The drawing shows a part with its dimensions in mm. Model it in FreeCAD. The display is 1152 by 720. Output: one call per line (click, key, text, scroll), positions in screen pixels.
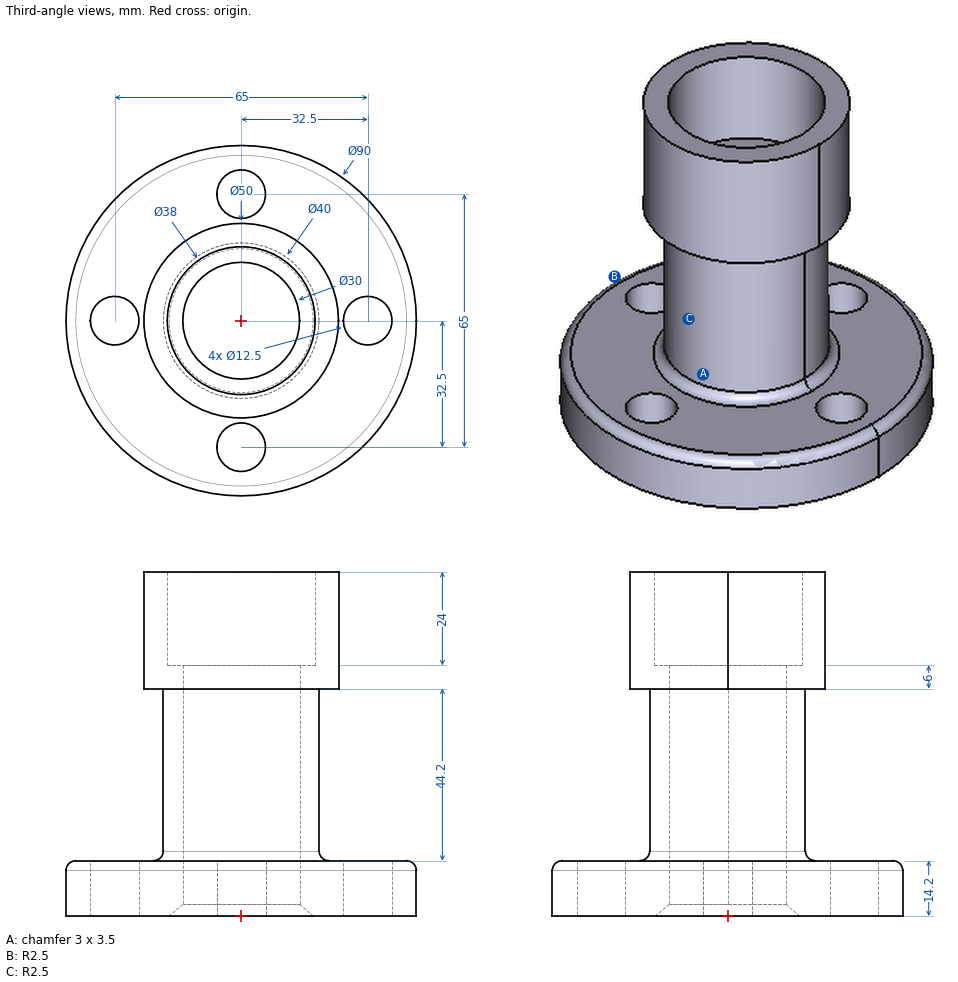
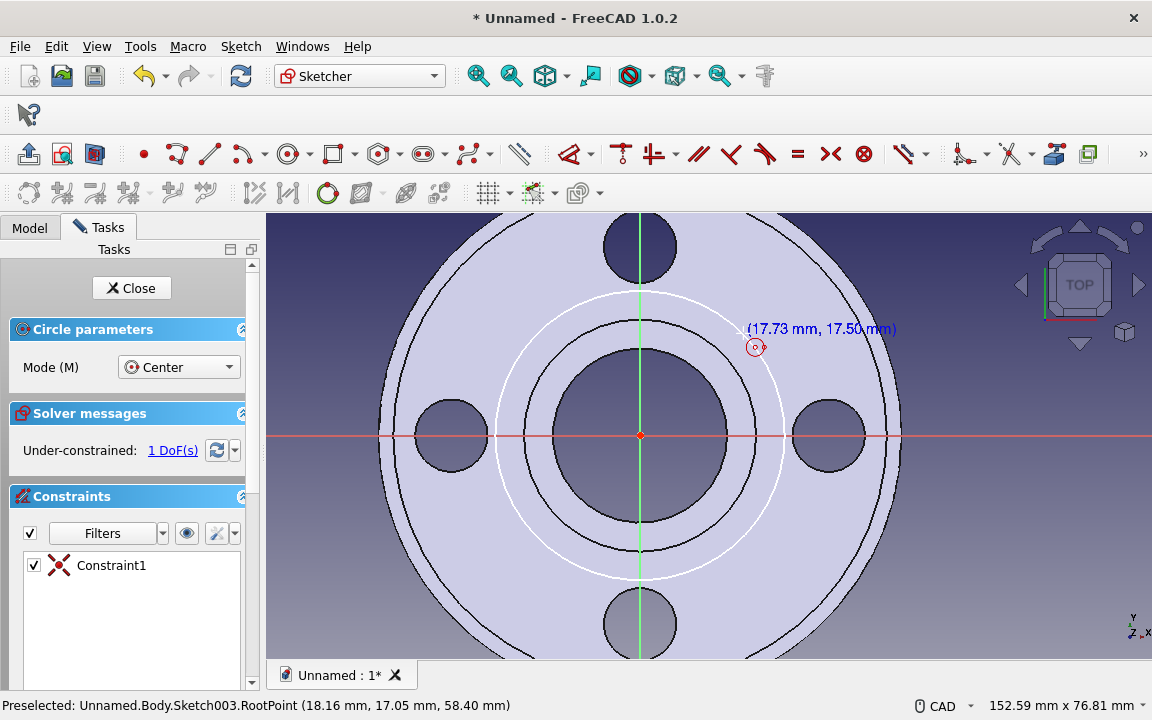
click(640, 436)
click(702, 374)
key(Escape)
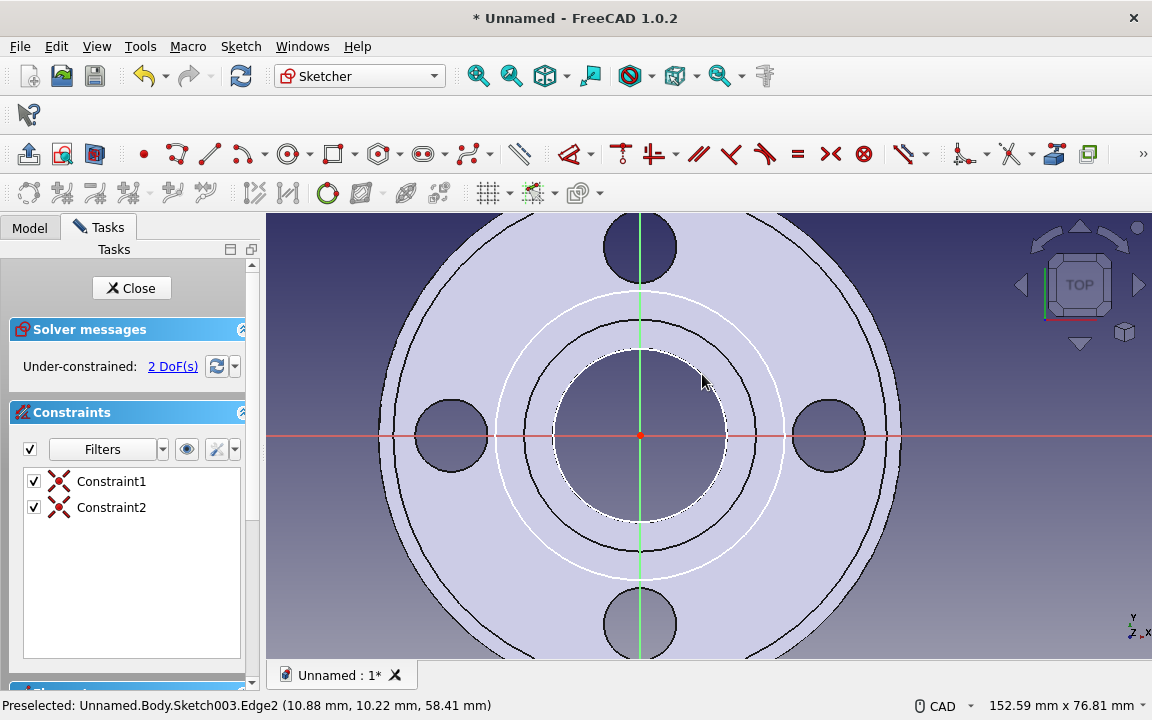
click(568, 154)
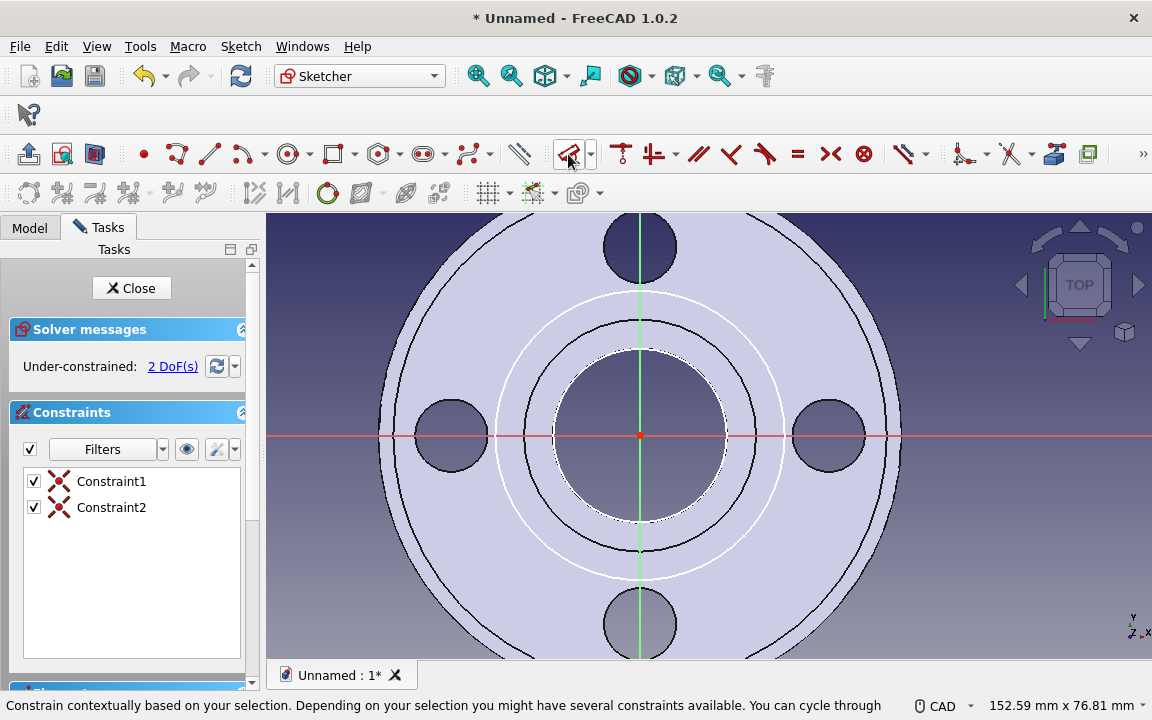
click(742, 333)
click(765, 310)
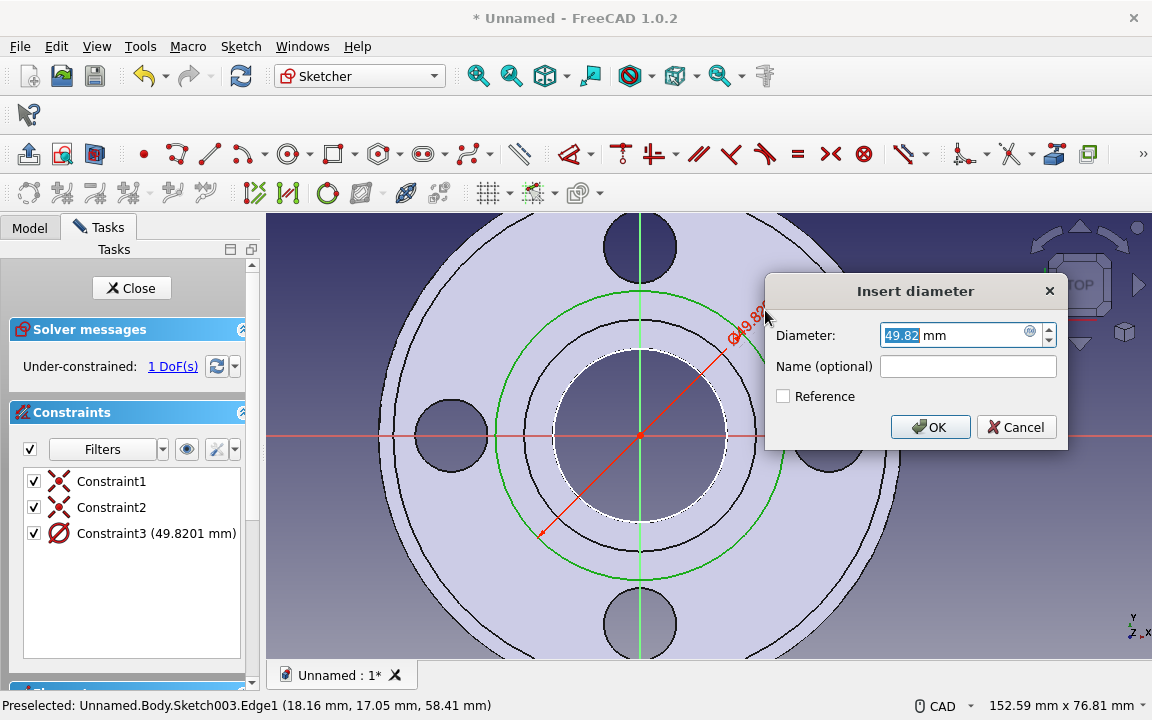
text(50)
key(Return)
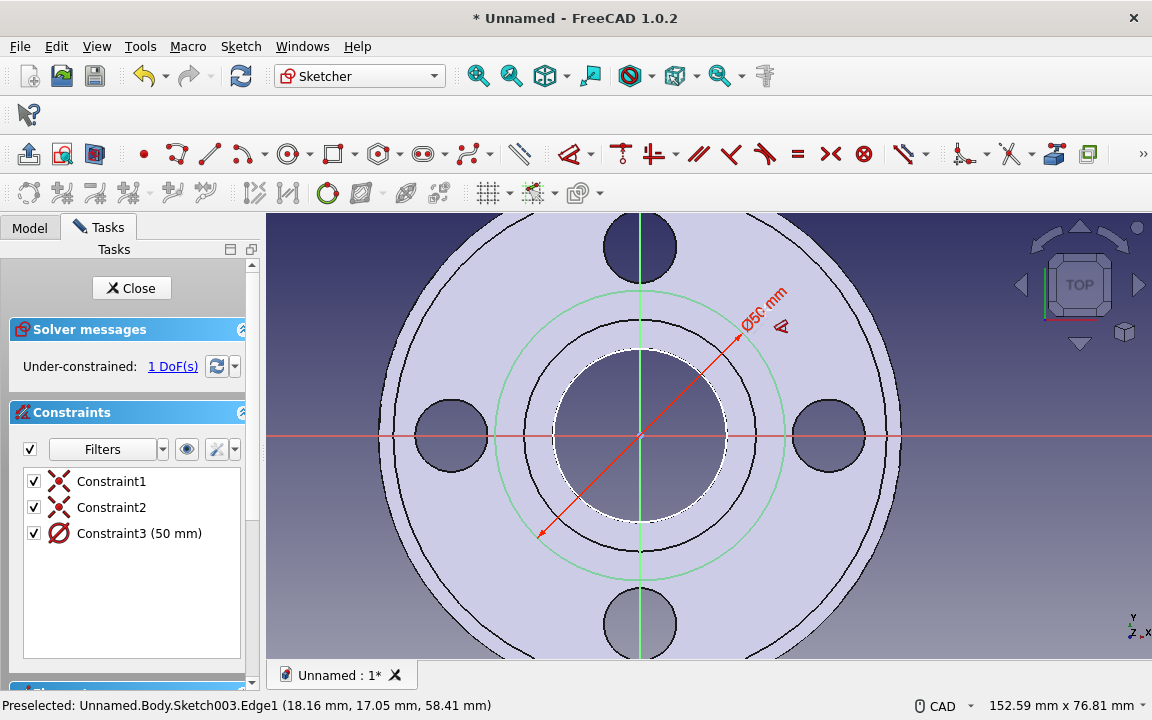
click(701, 374)
click(724, 351)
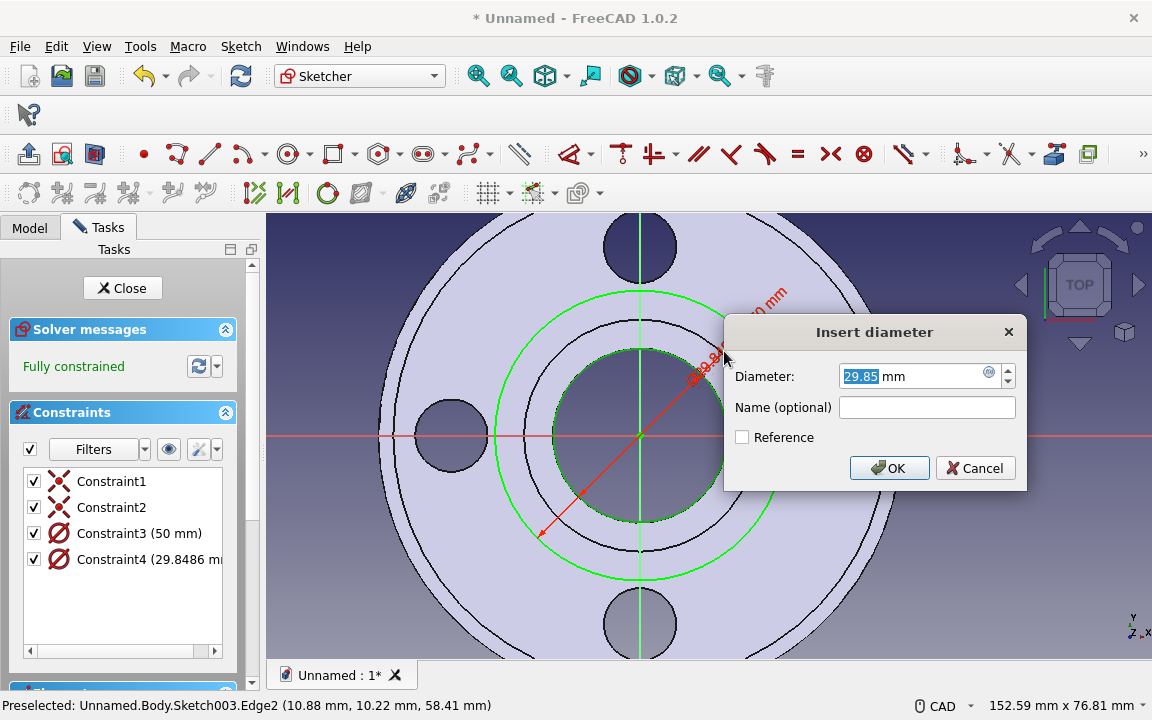
text(30)
key(Return)
key(Escape)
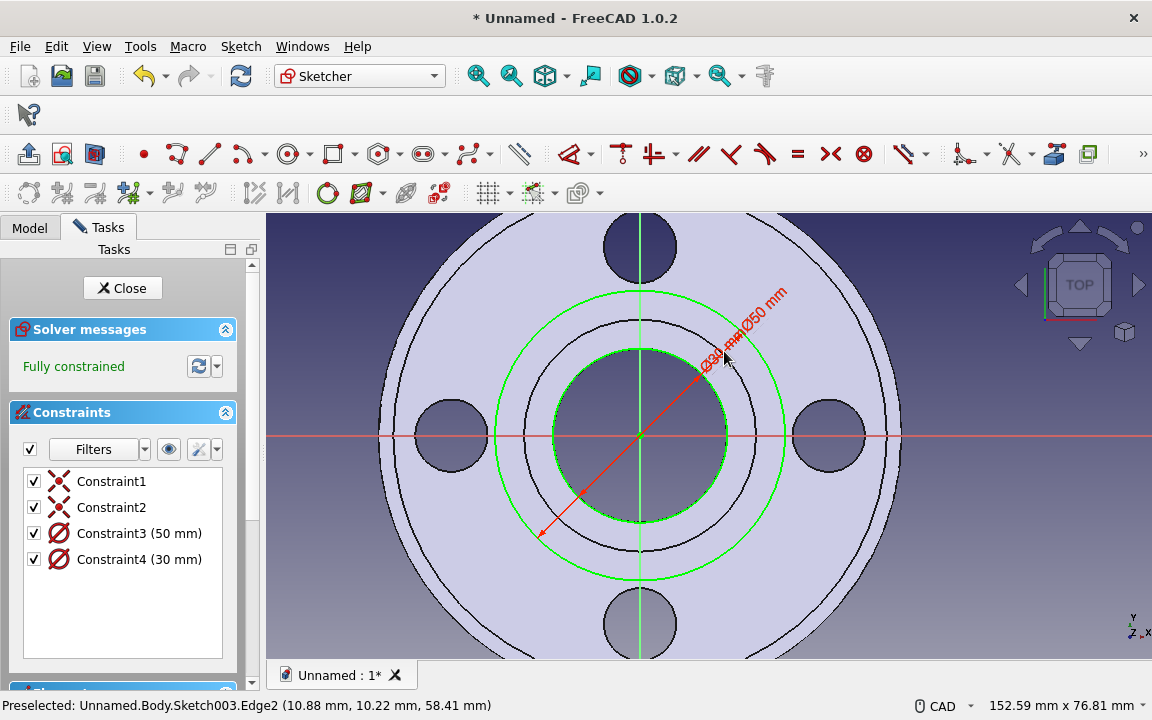
click(123, 288)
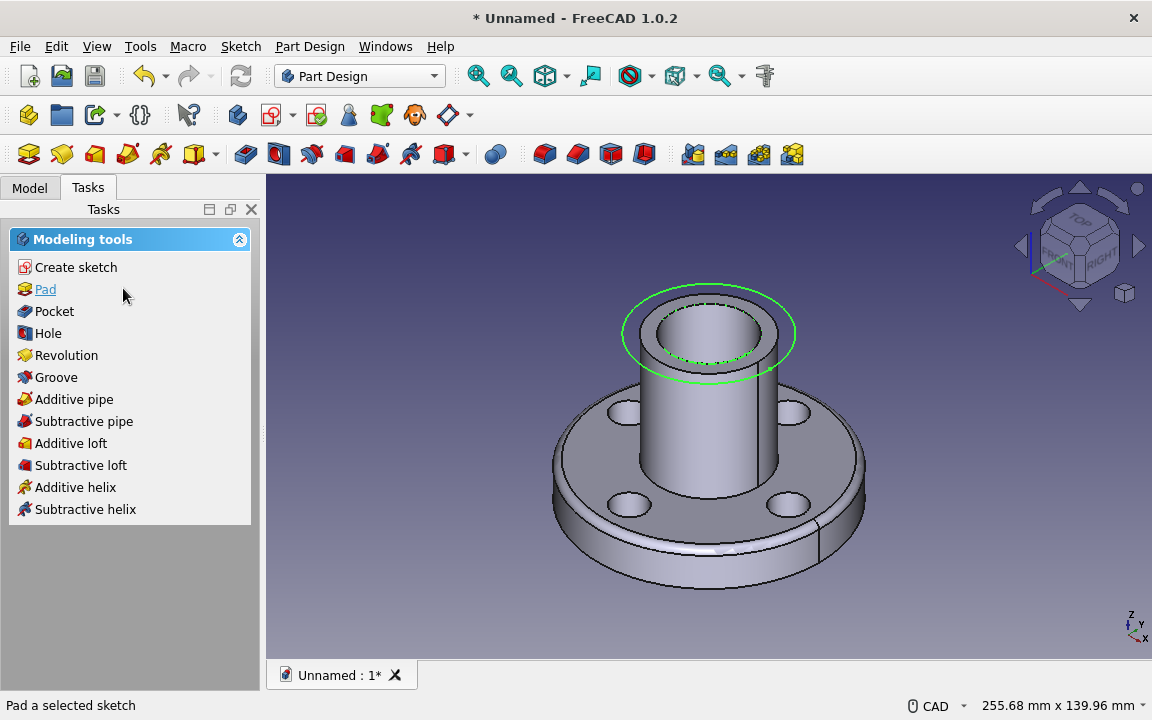
click(29, 154)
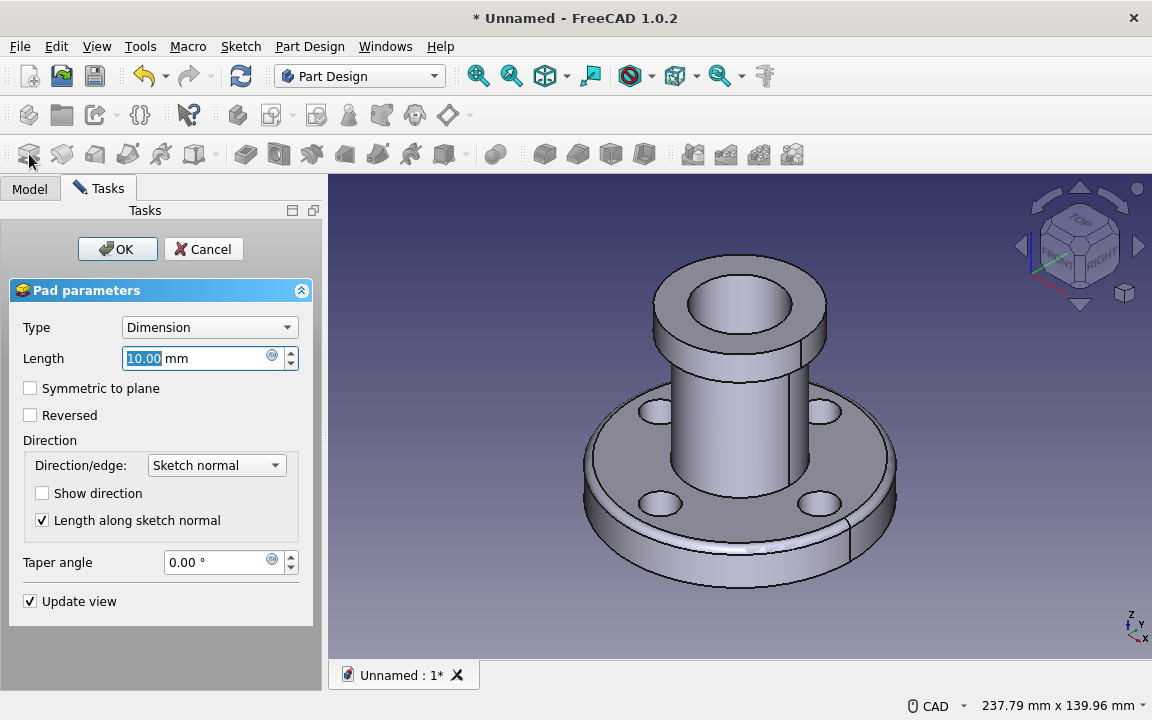
text(6)
key(Tab)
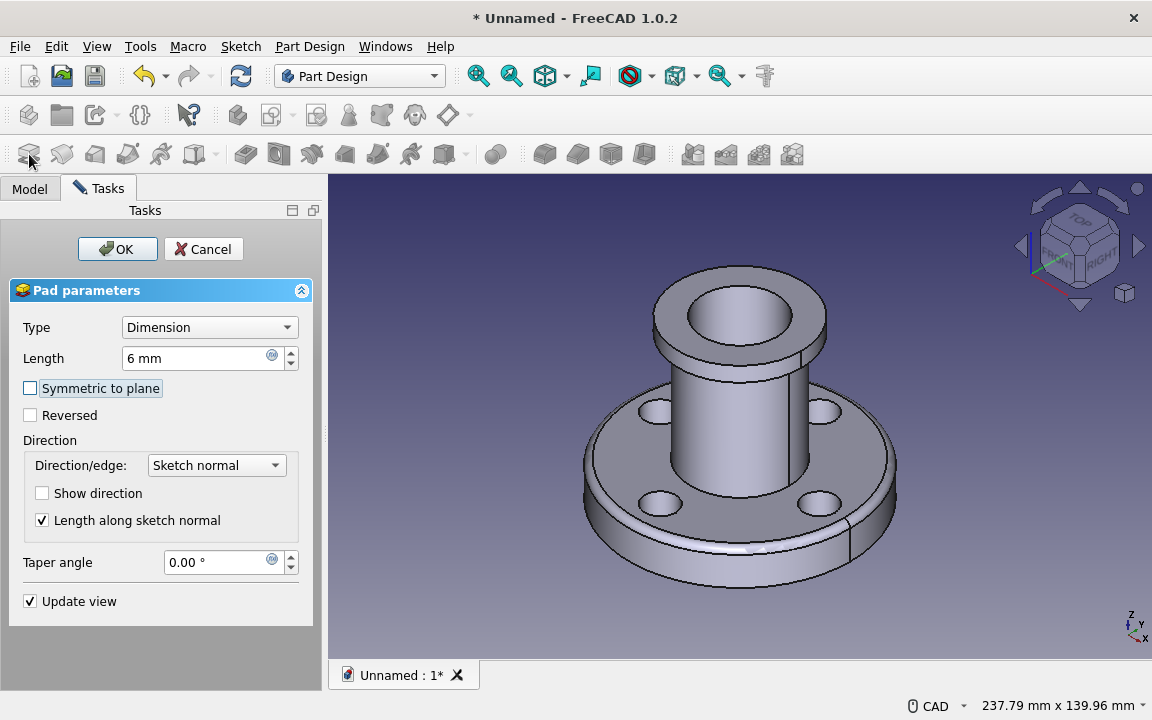
click(118, 249)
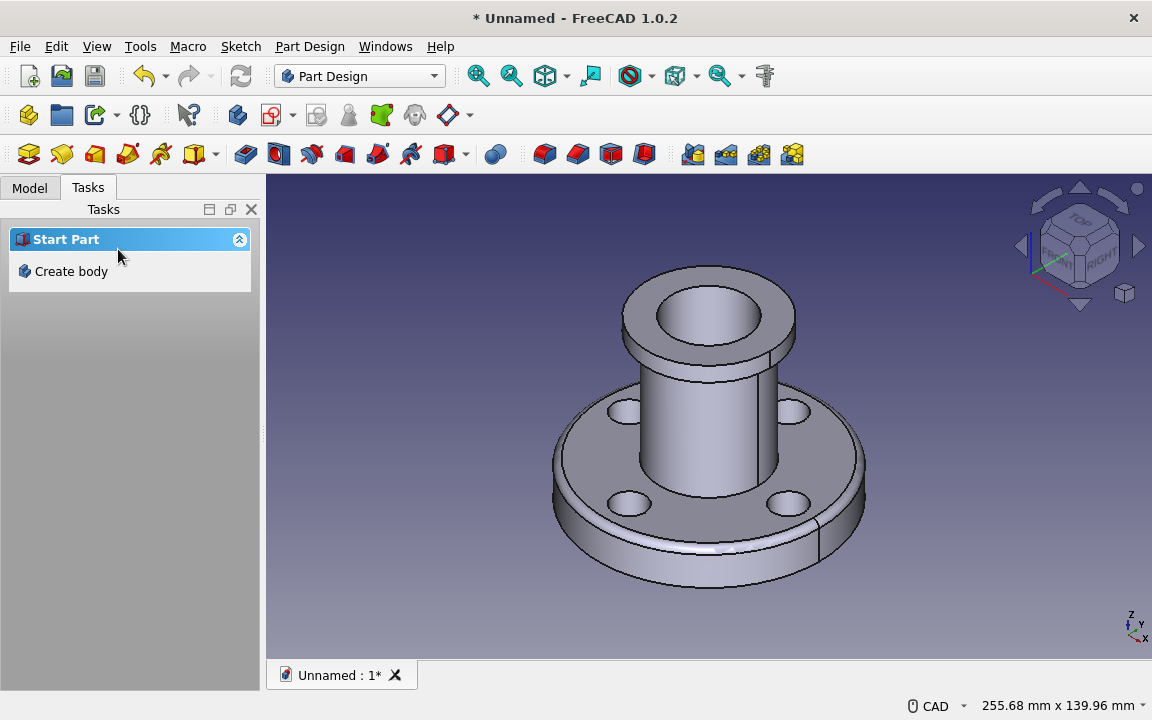
click(709, 355)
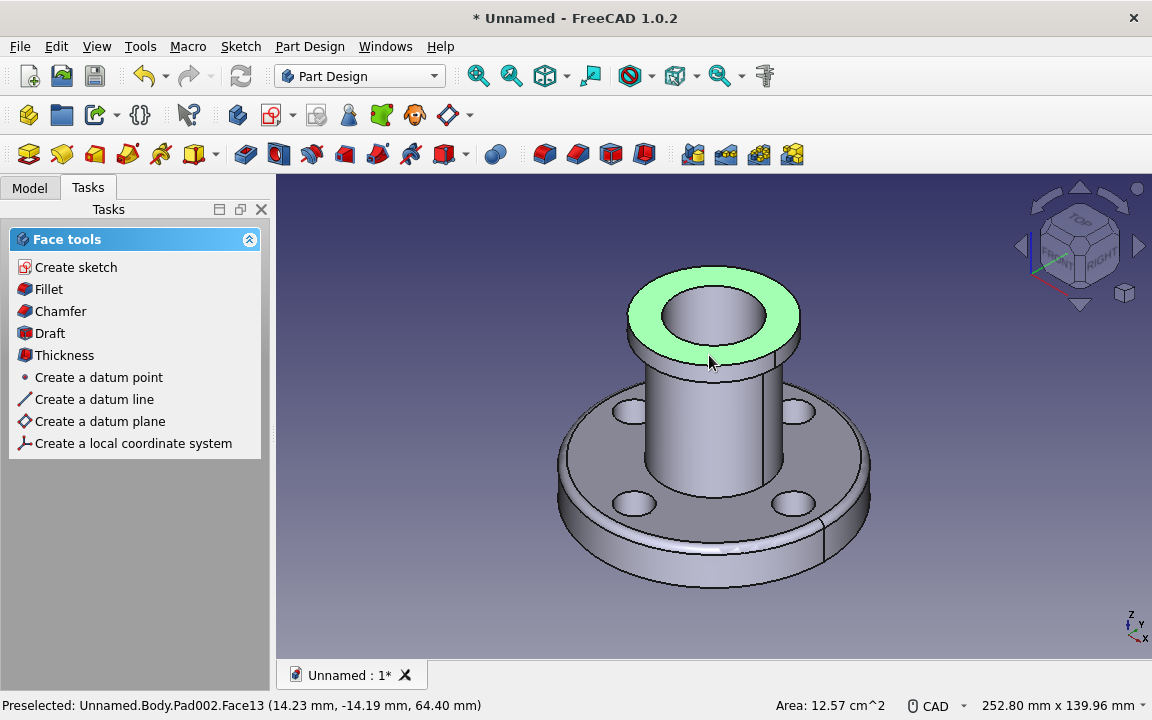
click(270, 116)